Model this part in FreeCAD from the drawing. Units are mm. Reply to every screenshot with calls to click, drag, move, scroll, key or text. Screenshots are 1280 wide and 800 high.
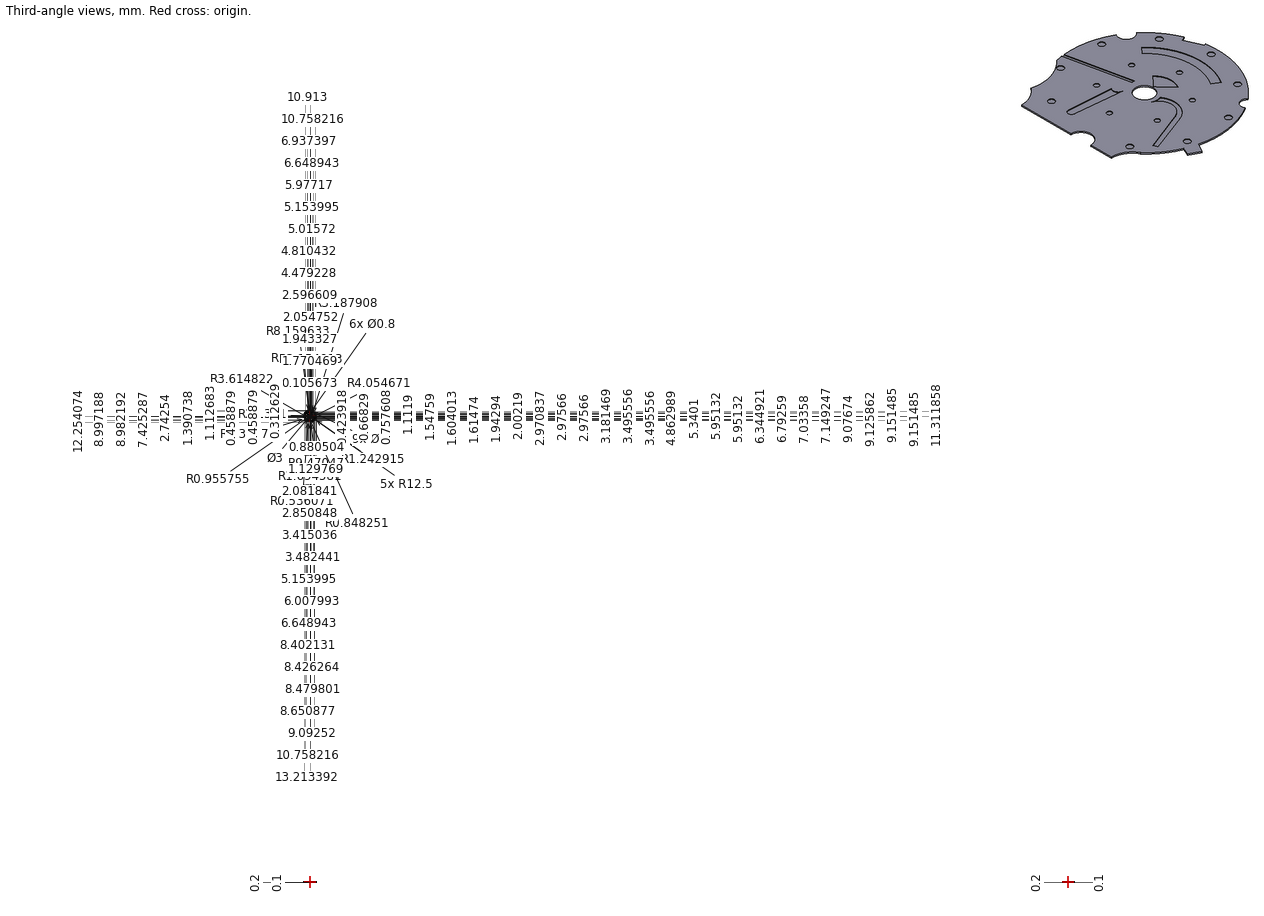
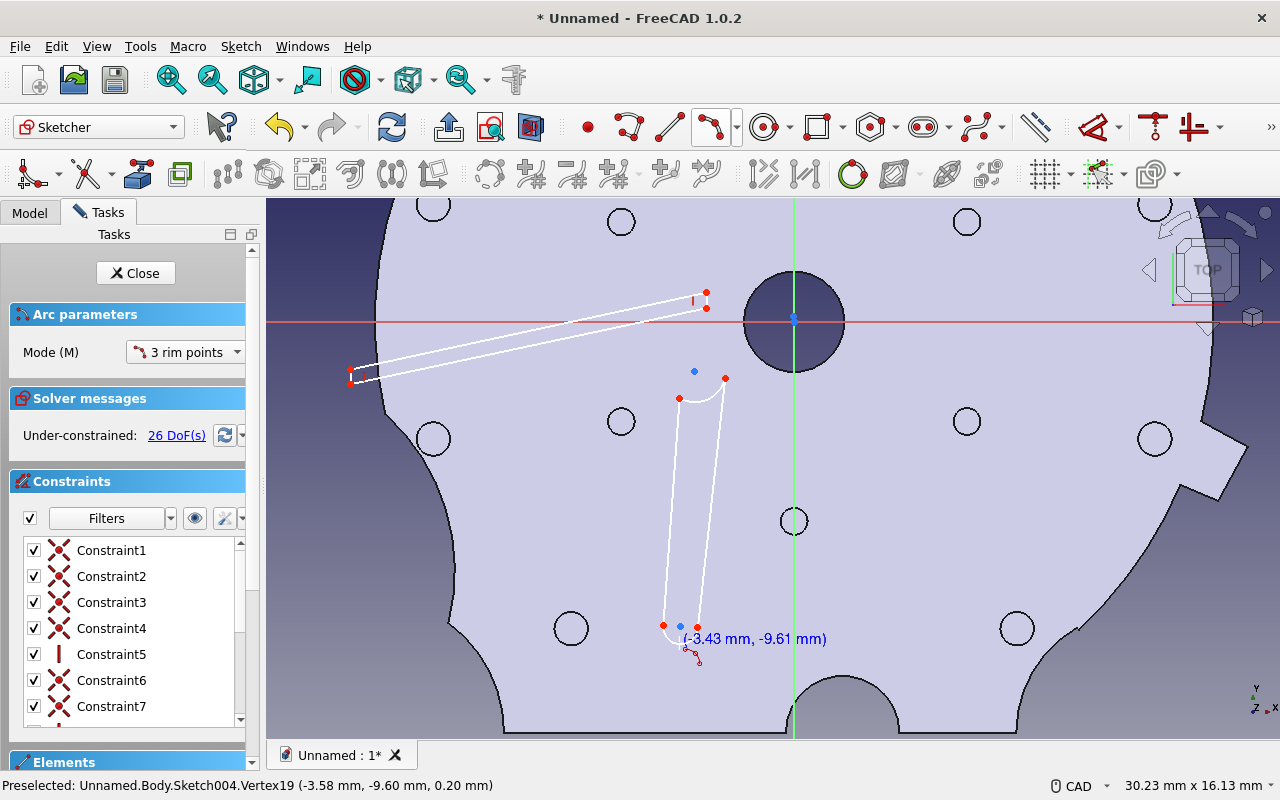
key(g)
key(m)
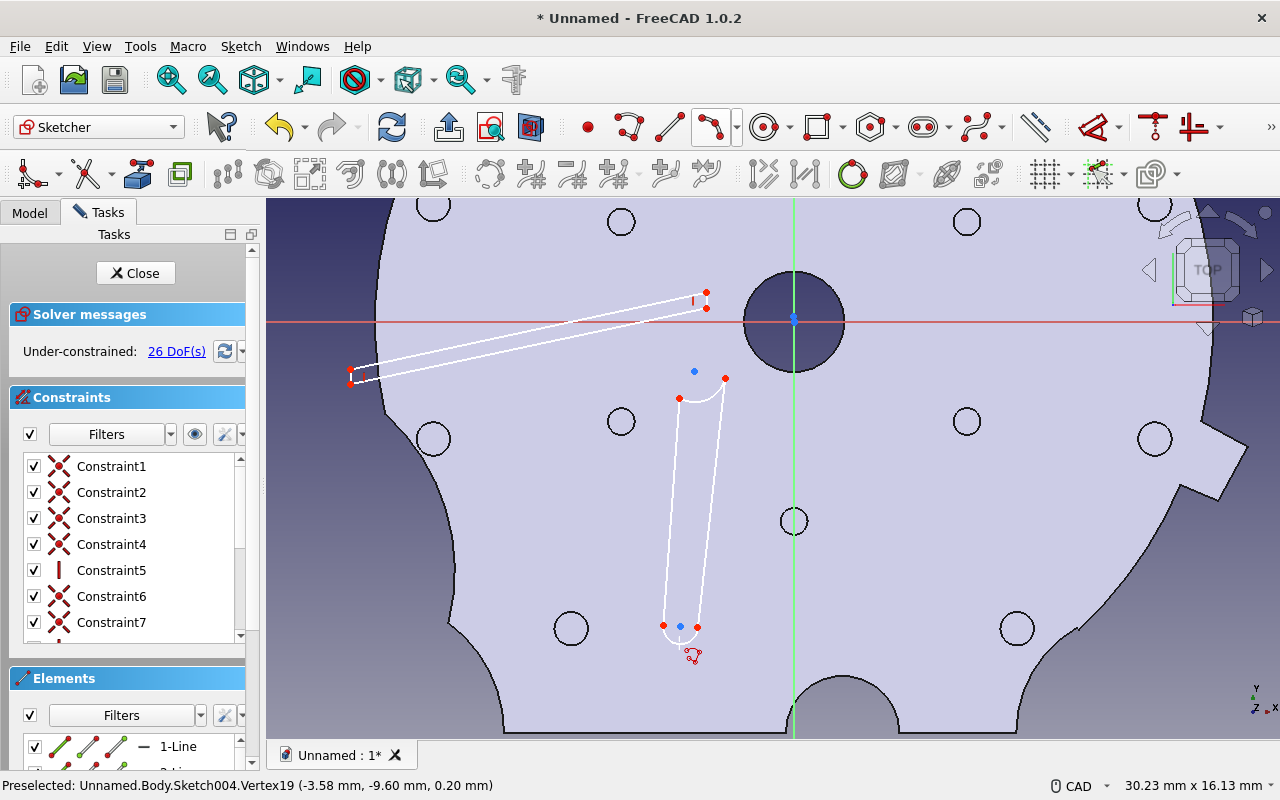
scroll(680, 643, down, 3)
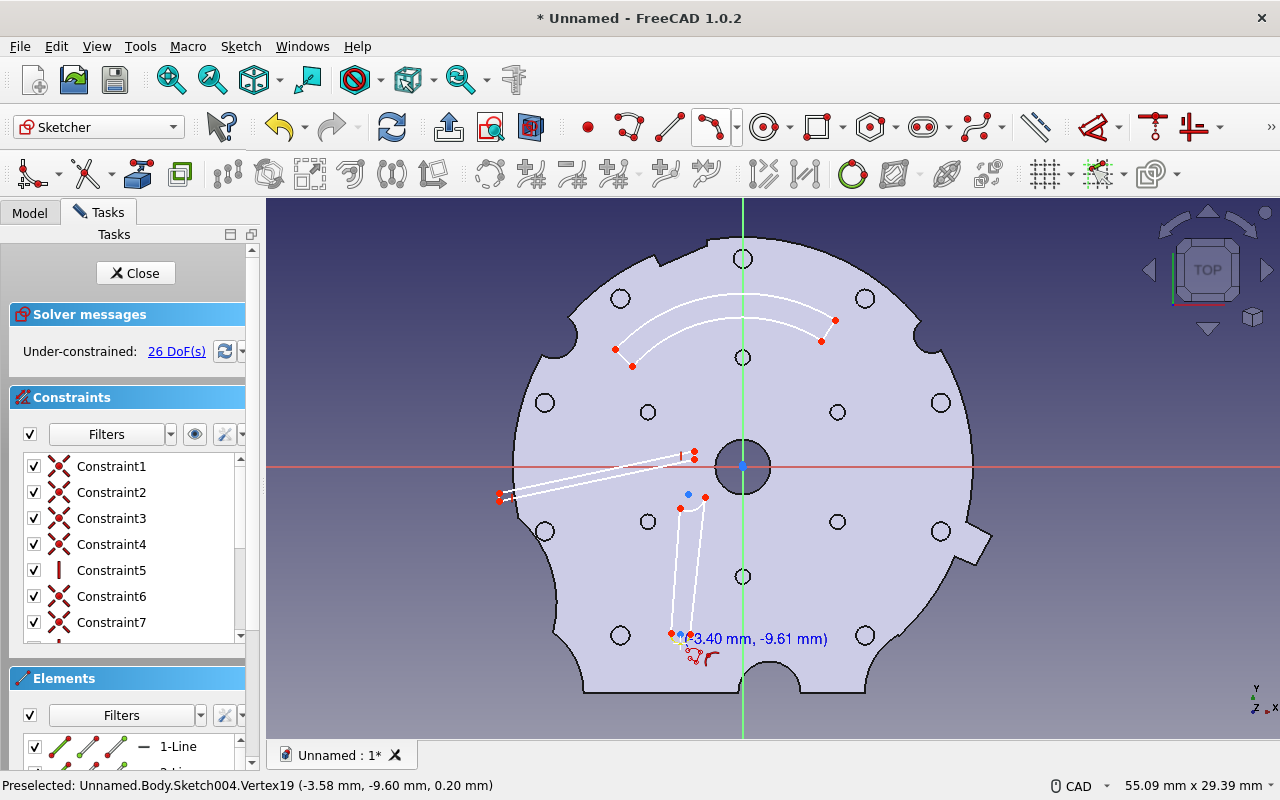
click(710, 409)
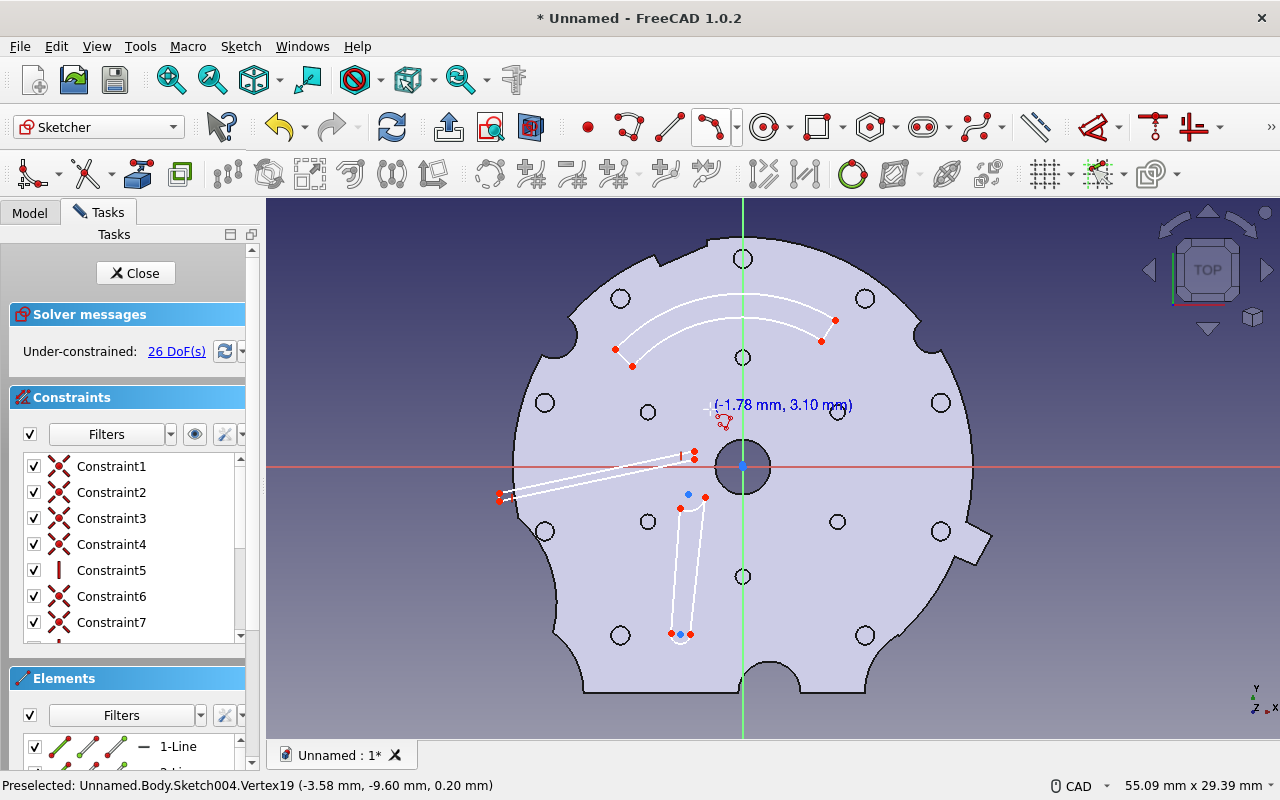
scroll(741, 437, up, 11)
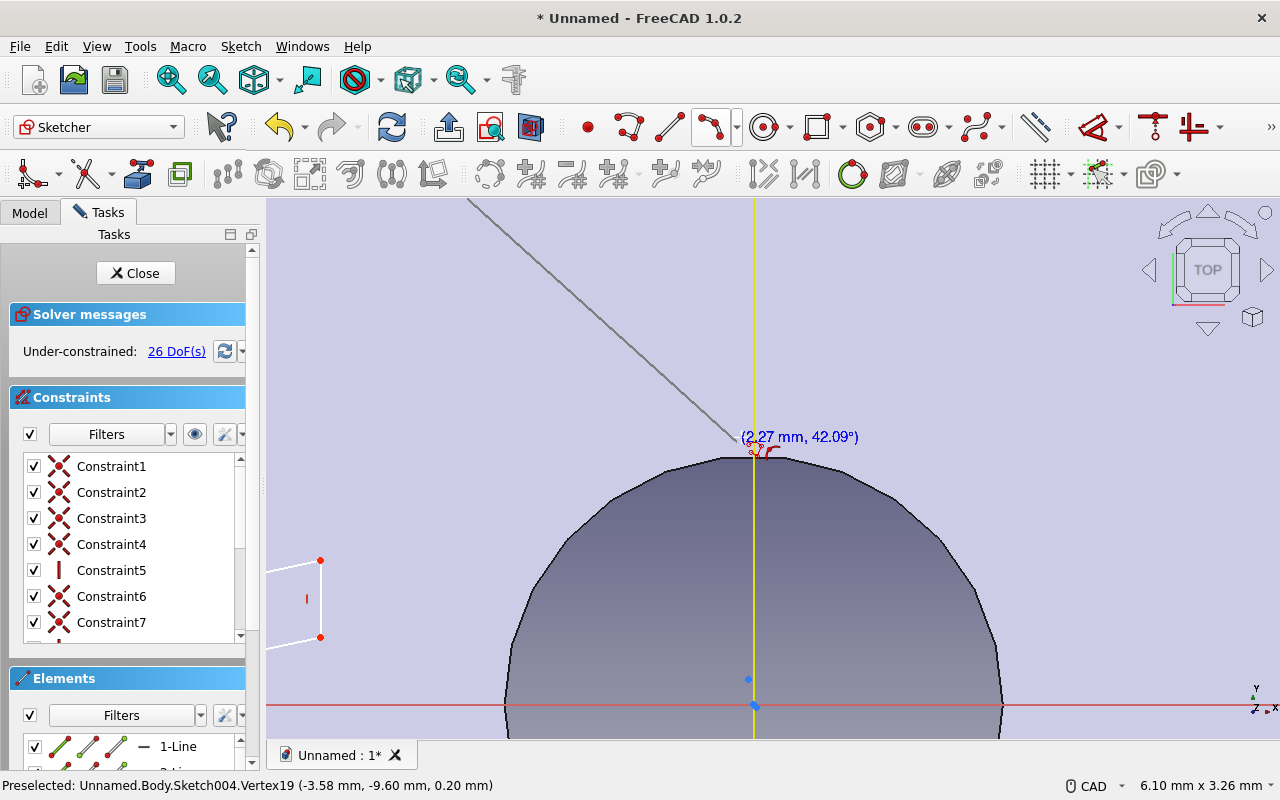
click(736, 434)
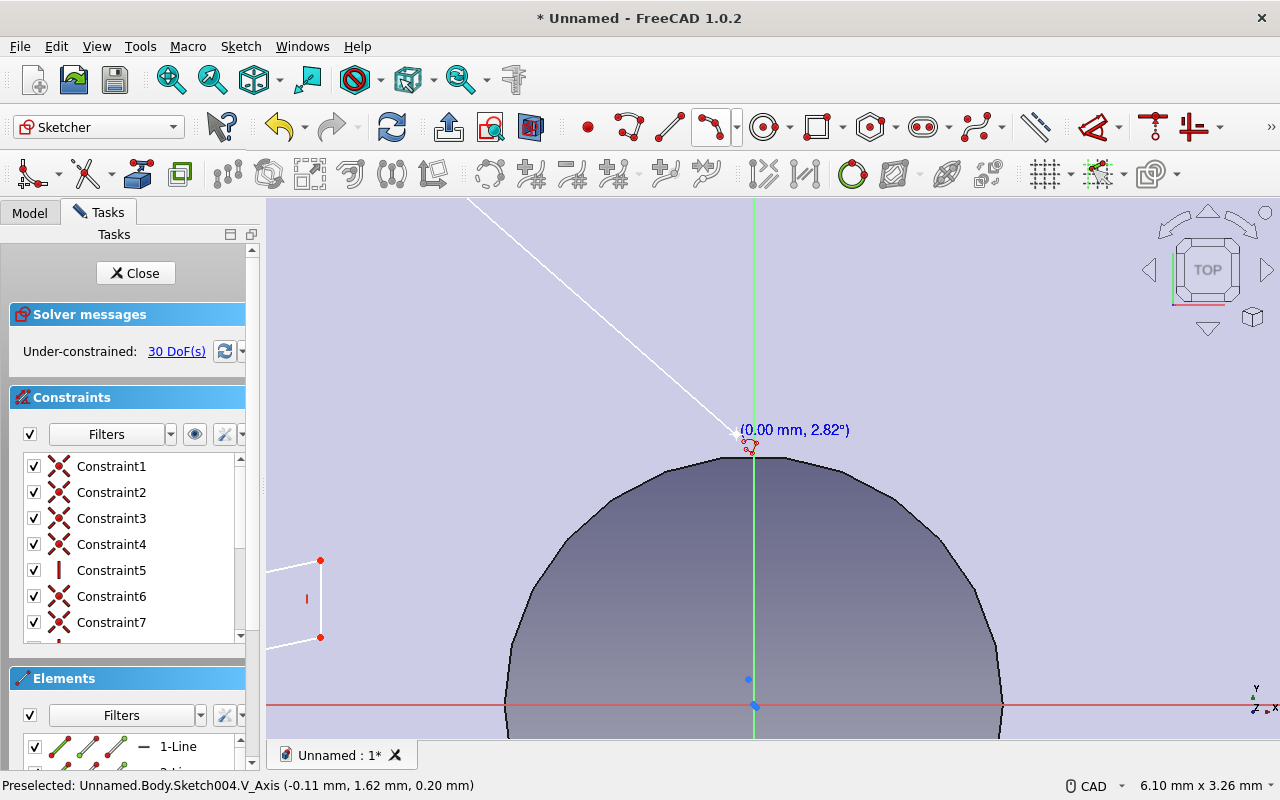
scroll(741, 437, down, 11)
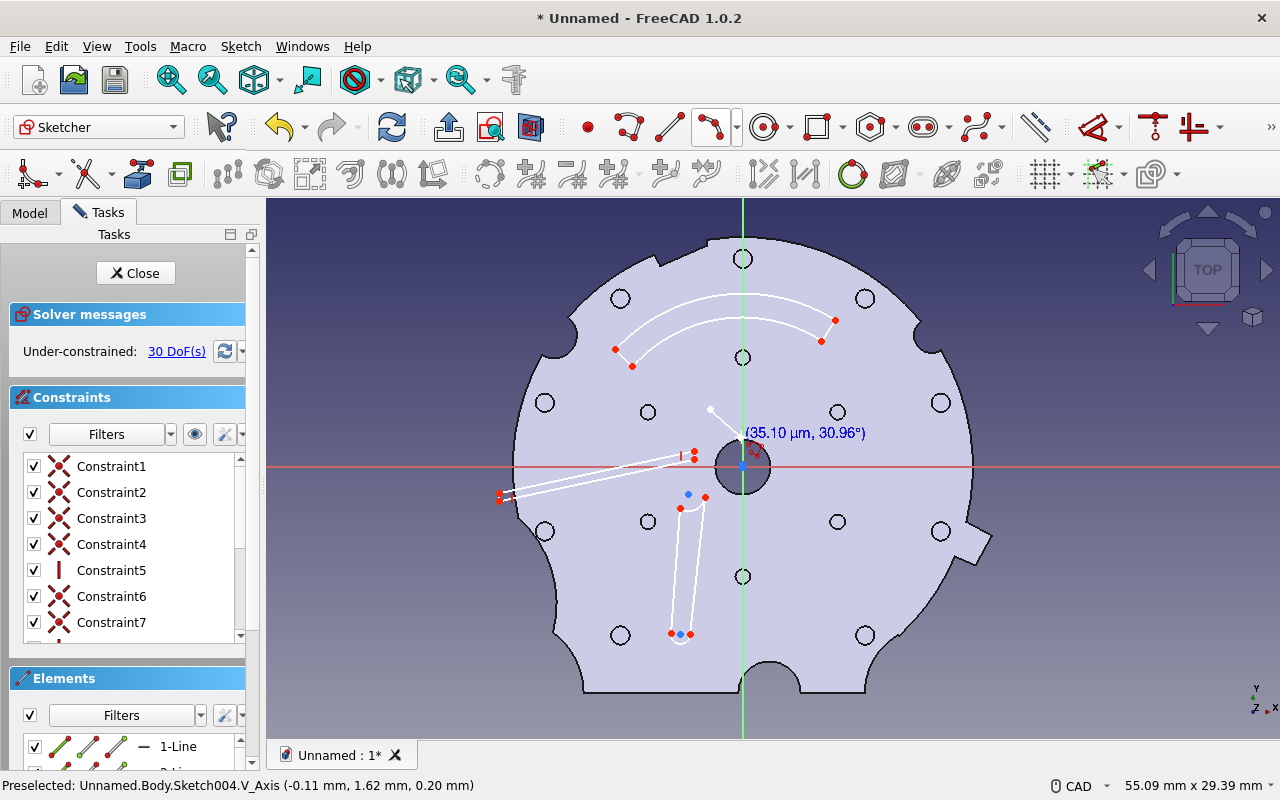
click(781, 400)
right_click(781, 400)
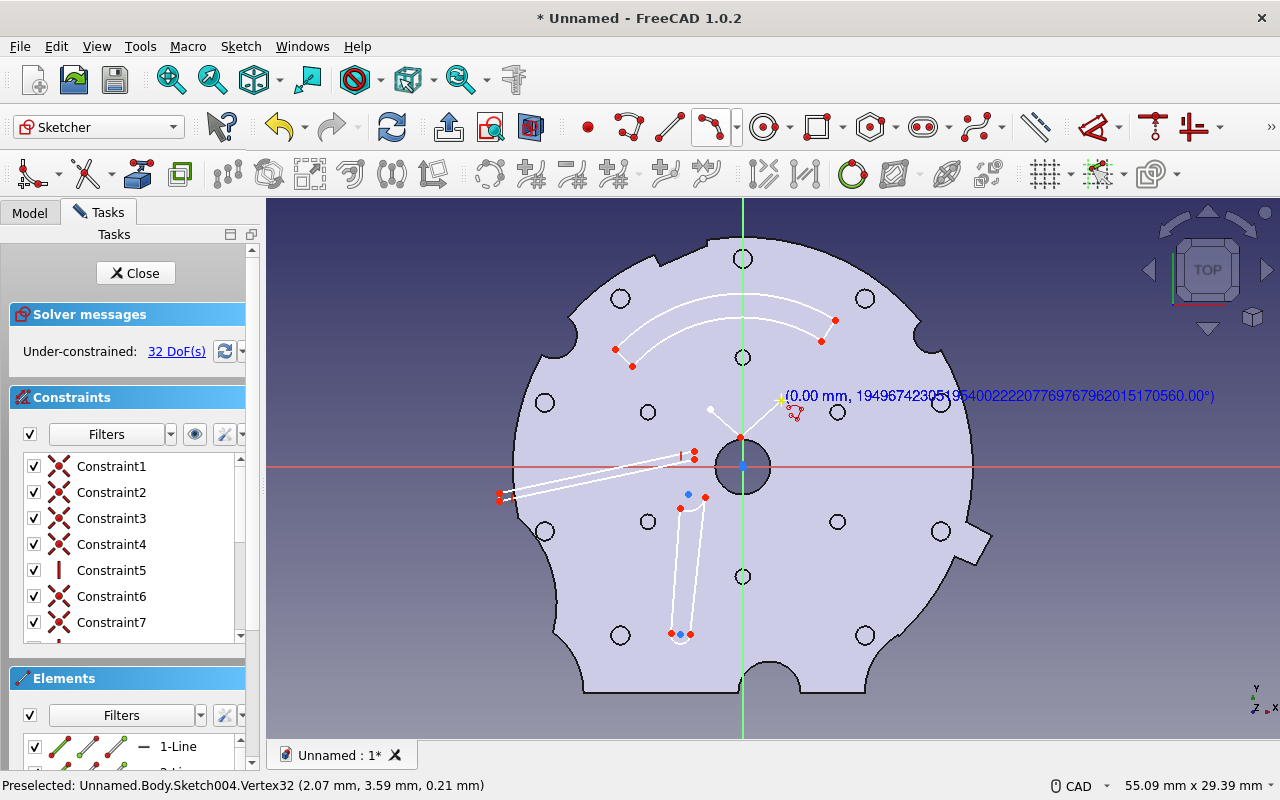
key(g)
key(3)
key(a)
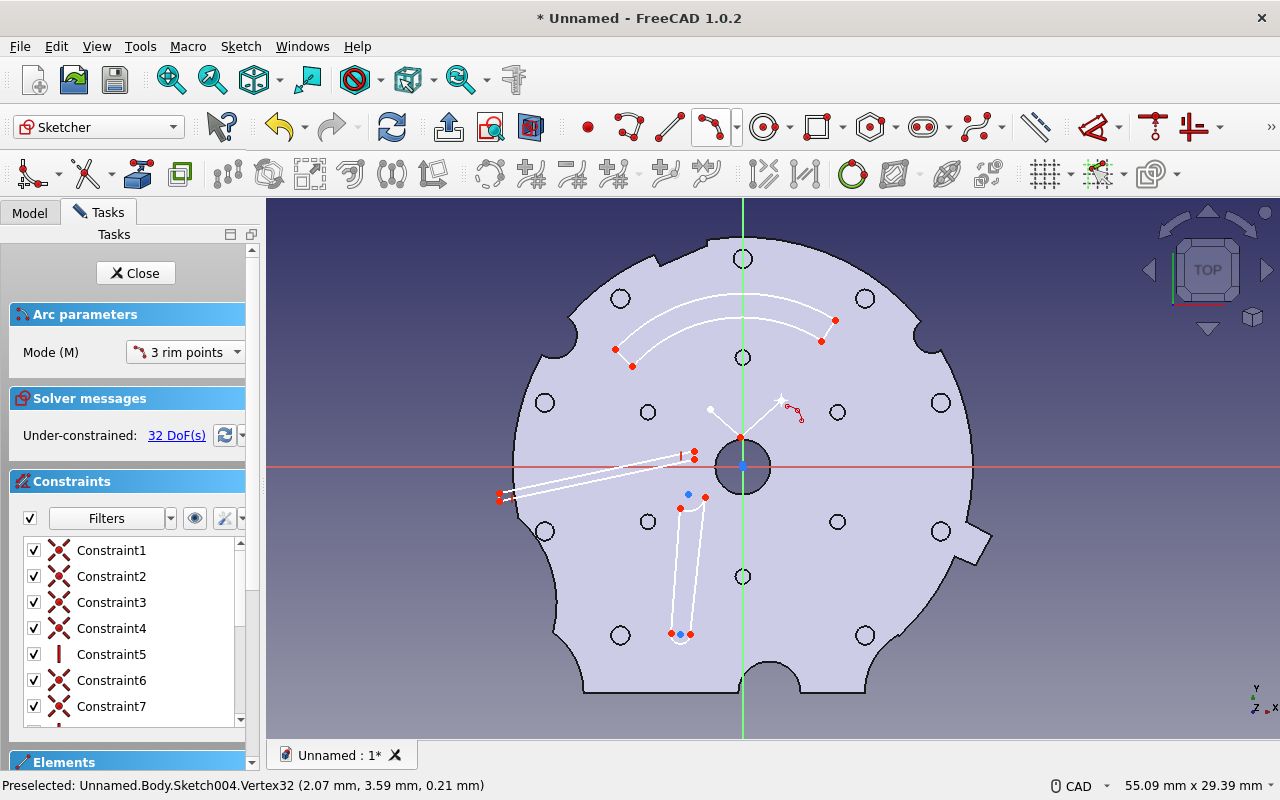
click(781, 401)
click(710, 410)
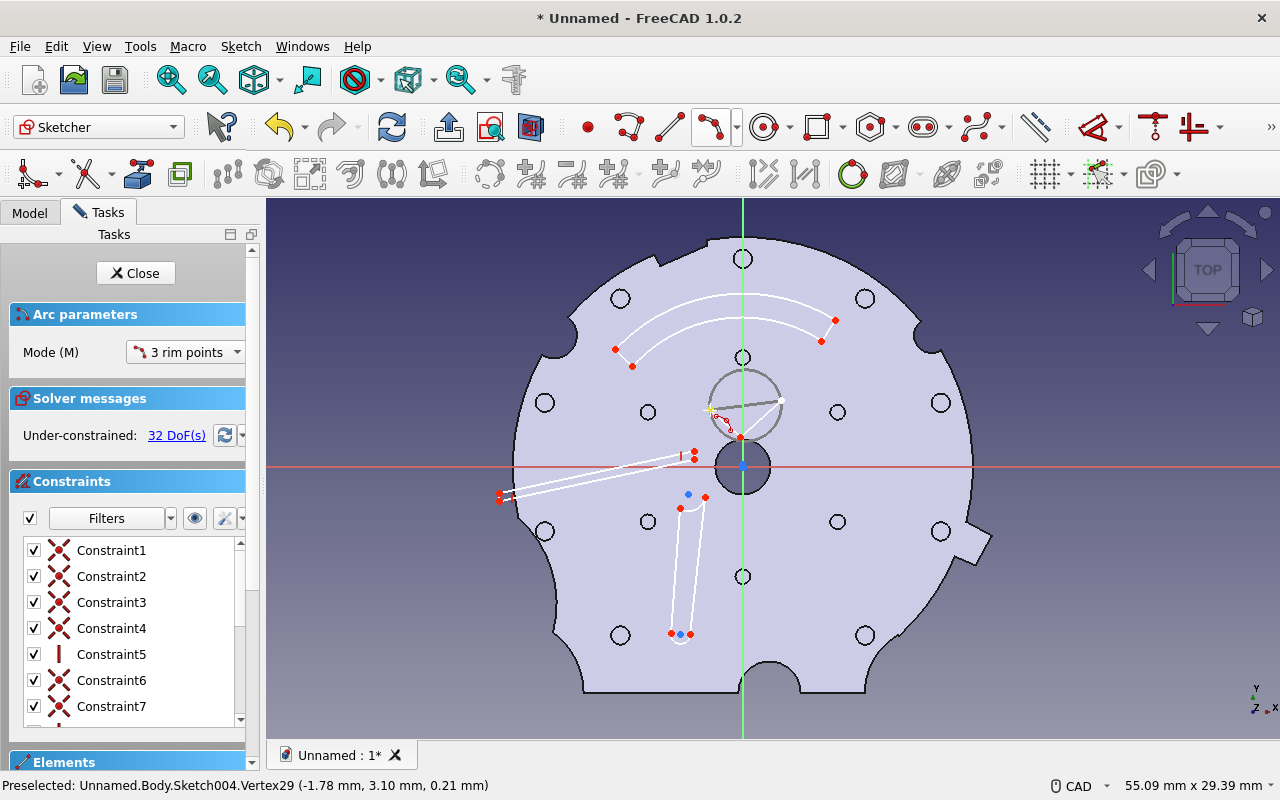
scroll(759, 392, up, 2)